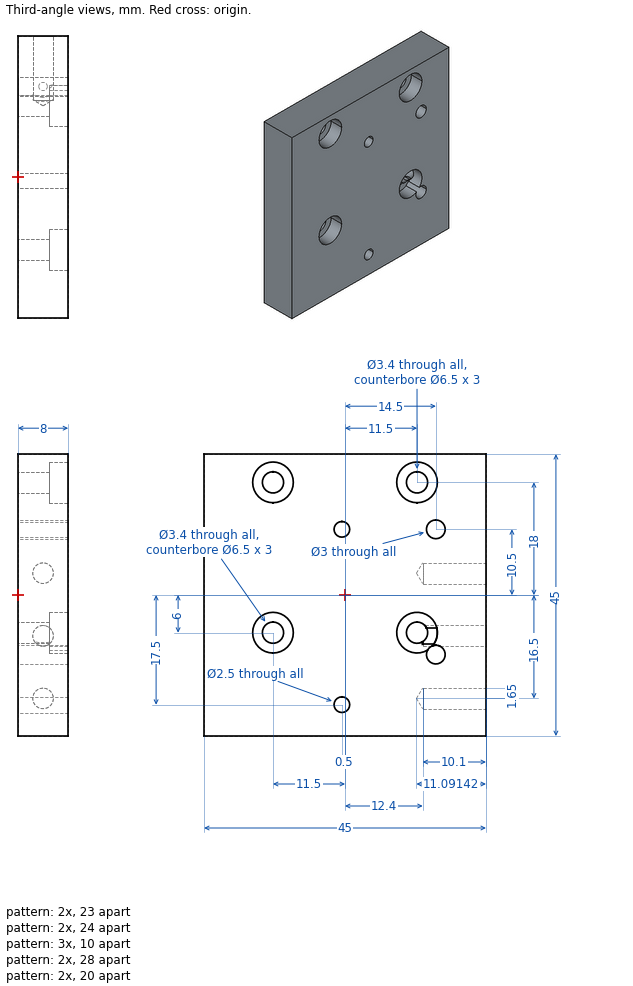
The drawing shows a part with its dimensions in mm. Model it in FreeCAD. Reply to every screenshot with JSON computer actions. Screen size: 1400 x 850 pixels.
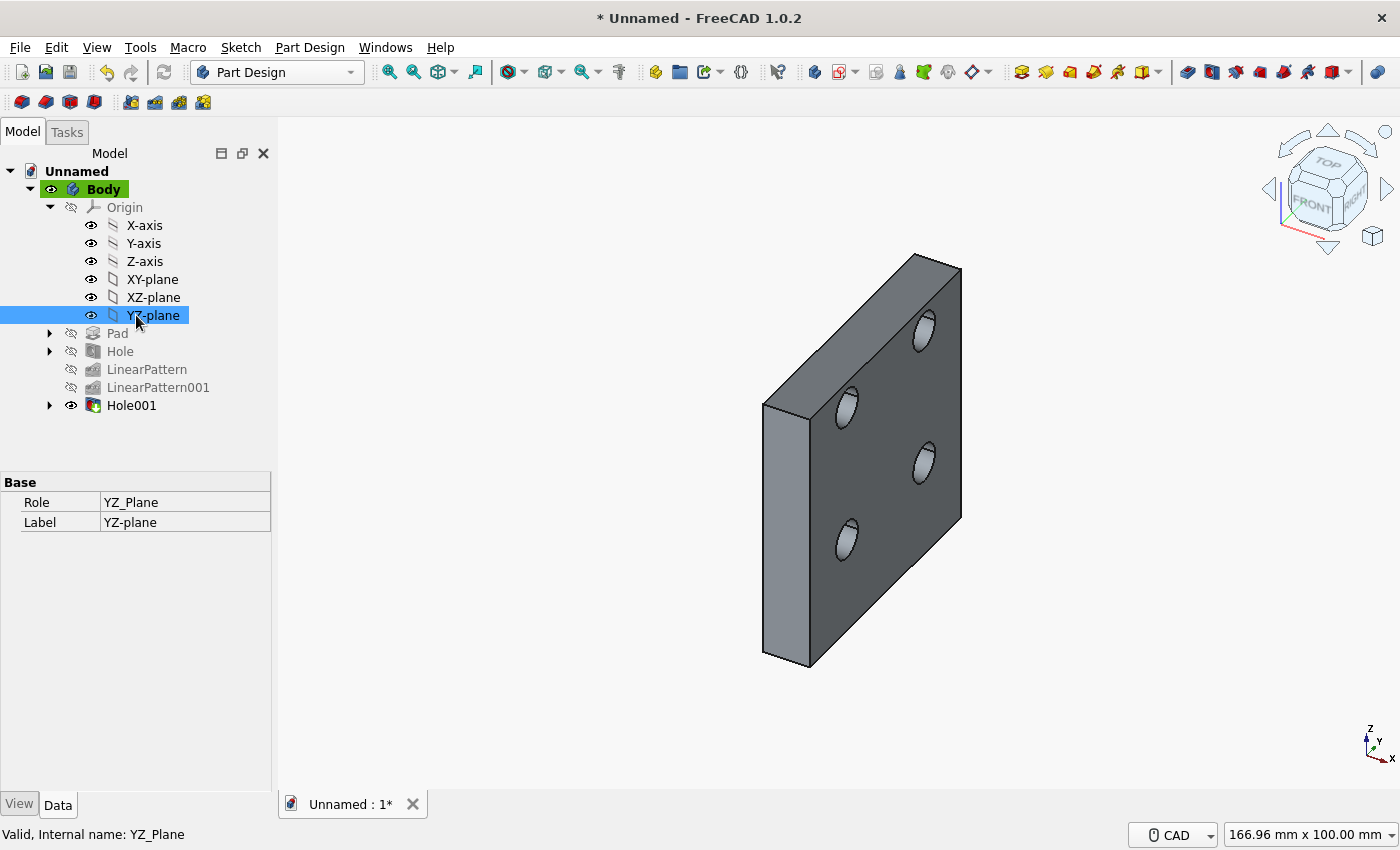
{"action": "left_click", "coordinate": [972, 72]}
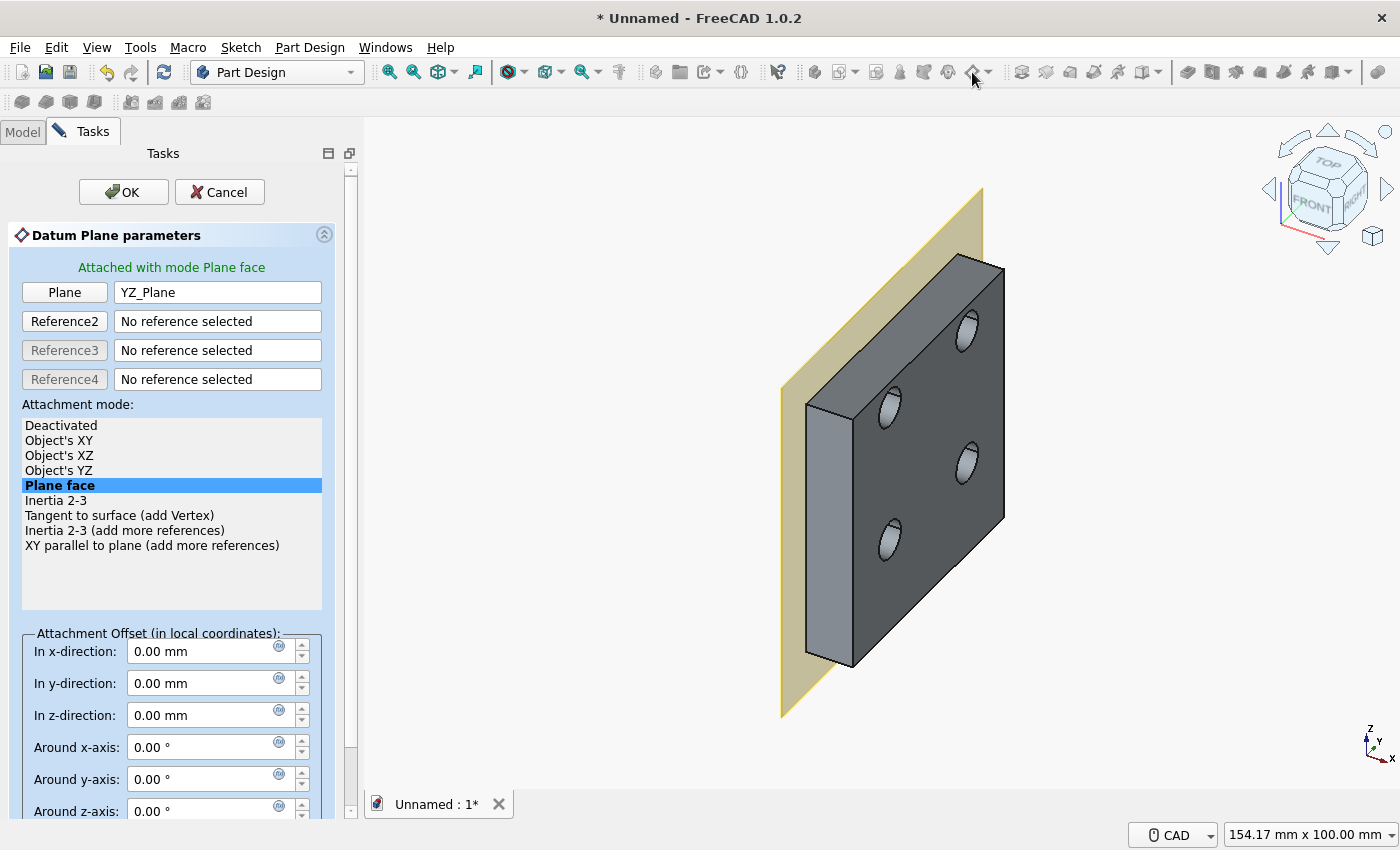
{"action": "triple_click", "coordinate": [210, 715]}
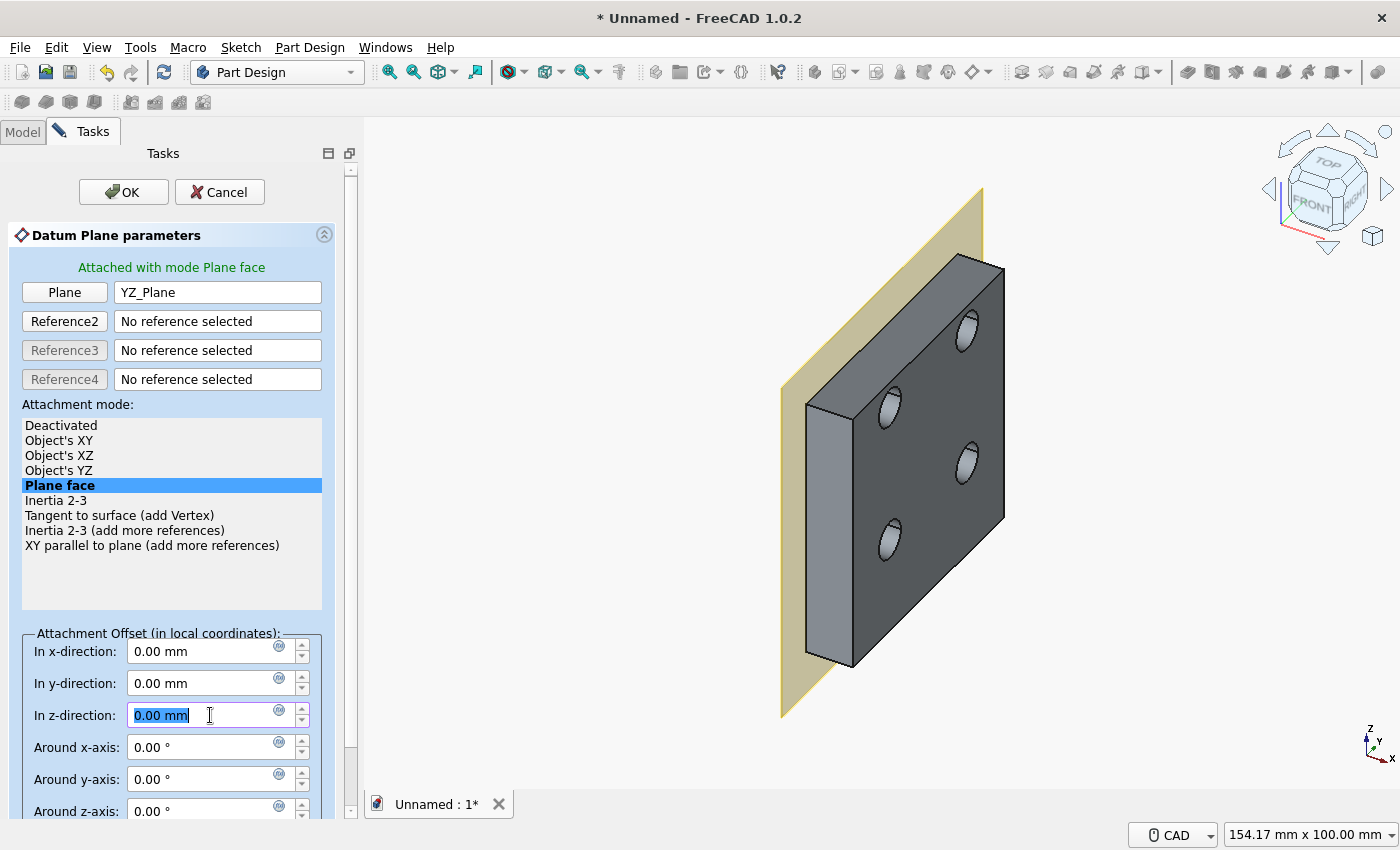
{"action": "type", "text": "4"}
{"action": "key", "text": "Tab"}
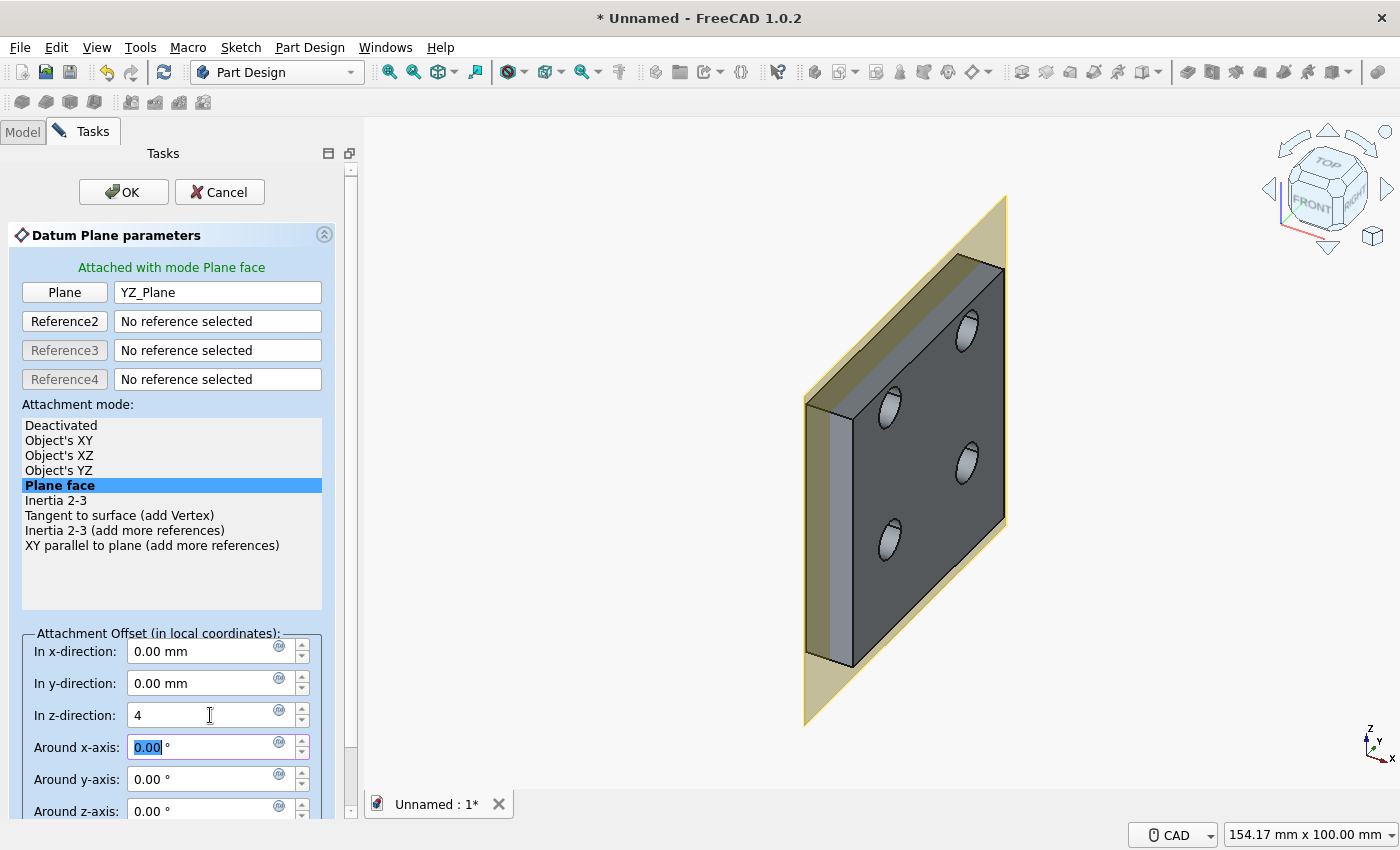
{"action": "left_click", "coordinate": [124, 192]}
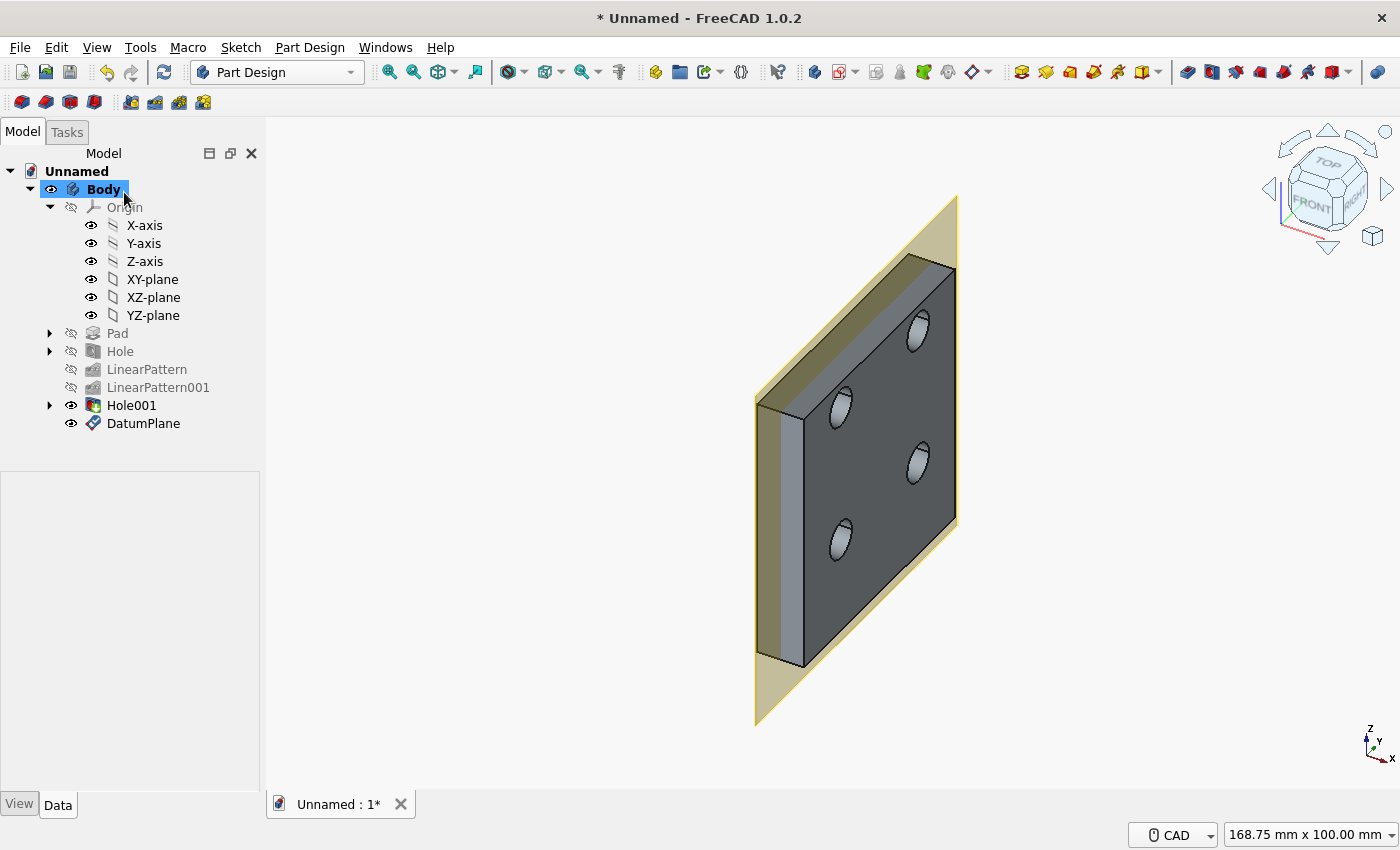
{"action": "left_click", "coordinate": [116, 423]}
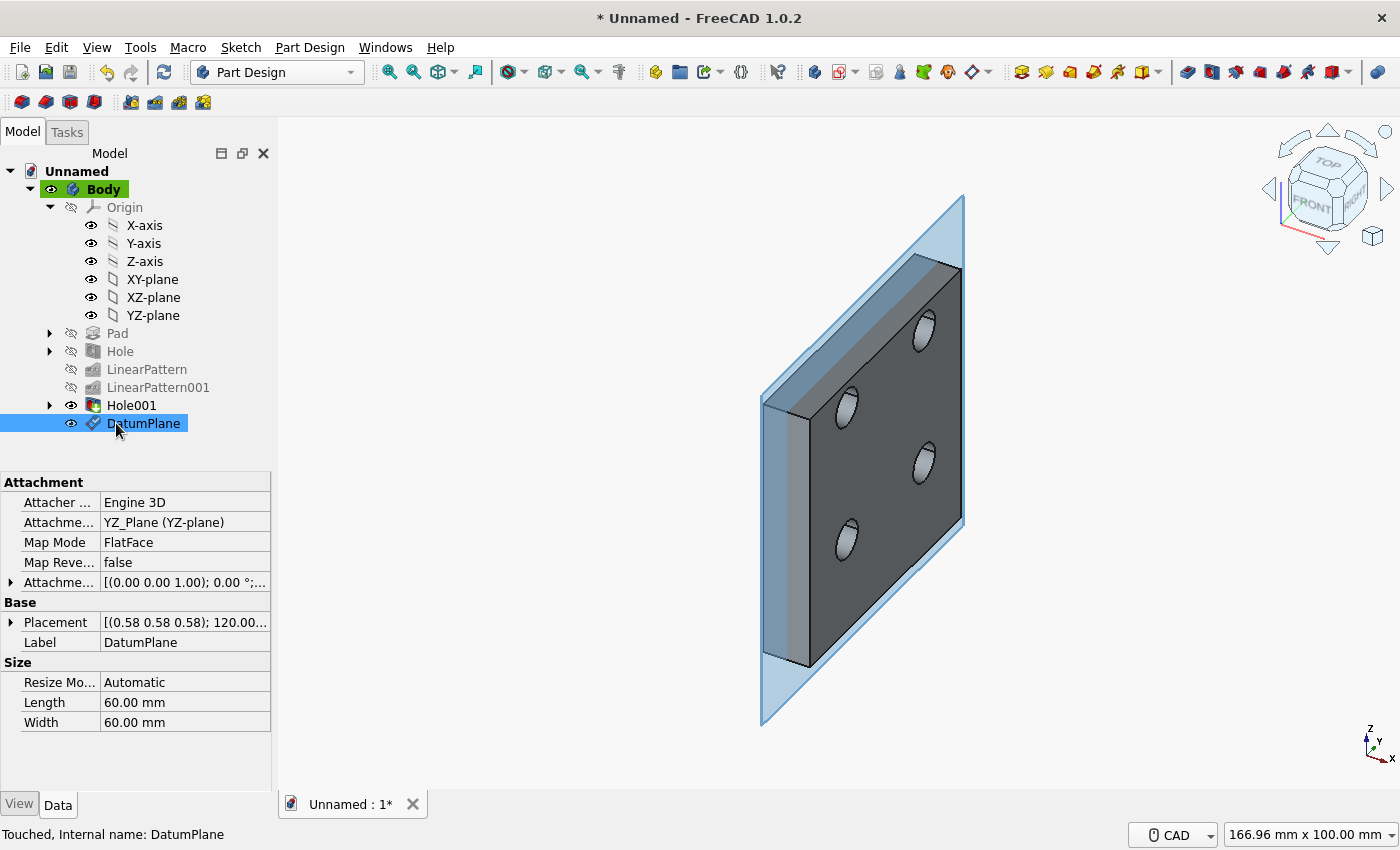
{"action": "left_click", "coordinate": [840, 72]}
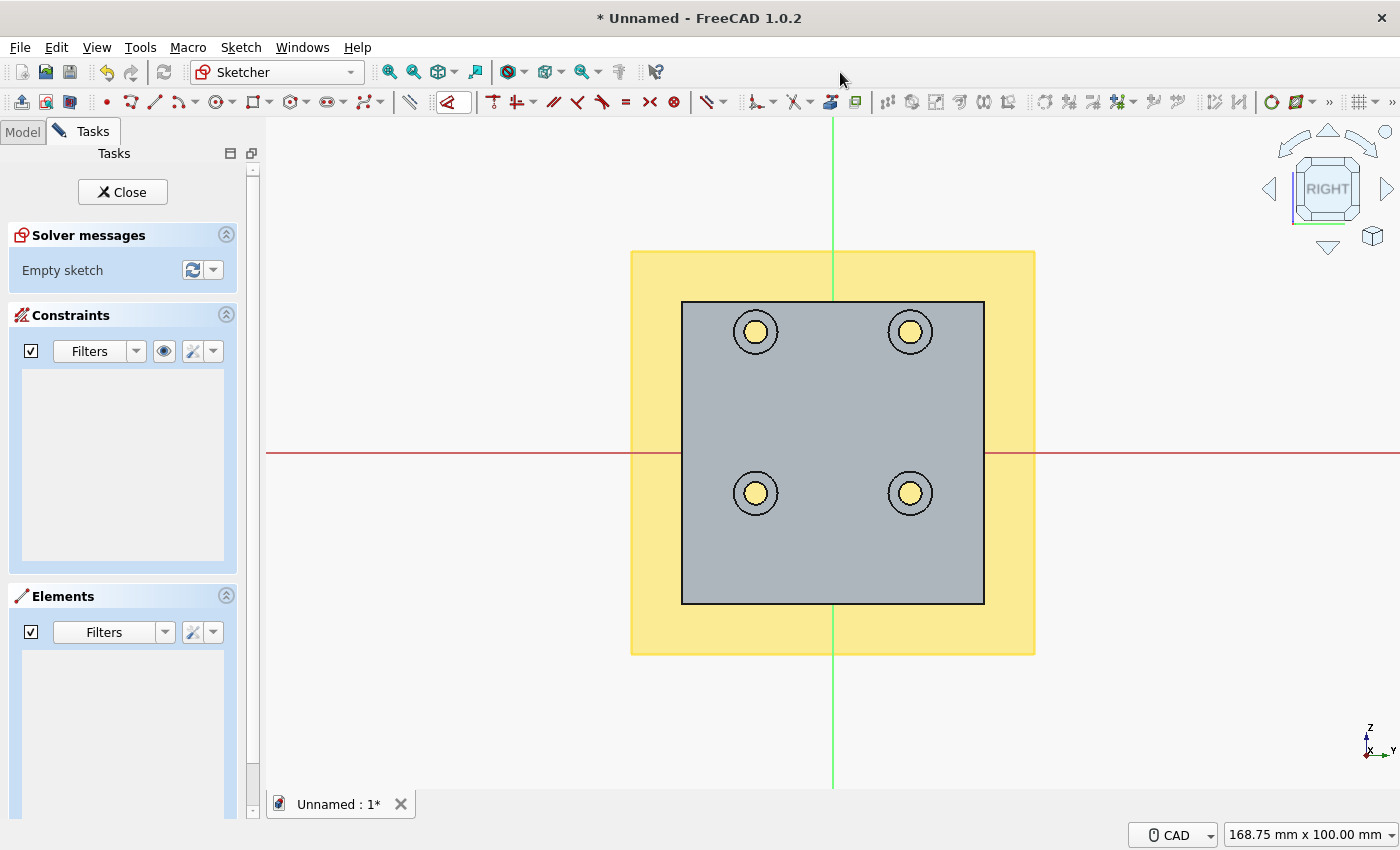
{"action": "key", "text": "q s"}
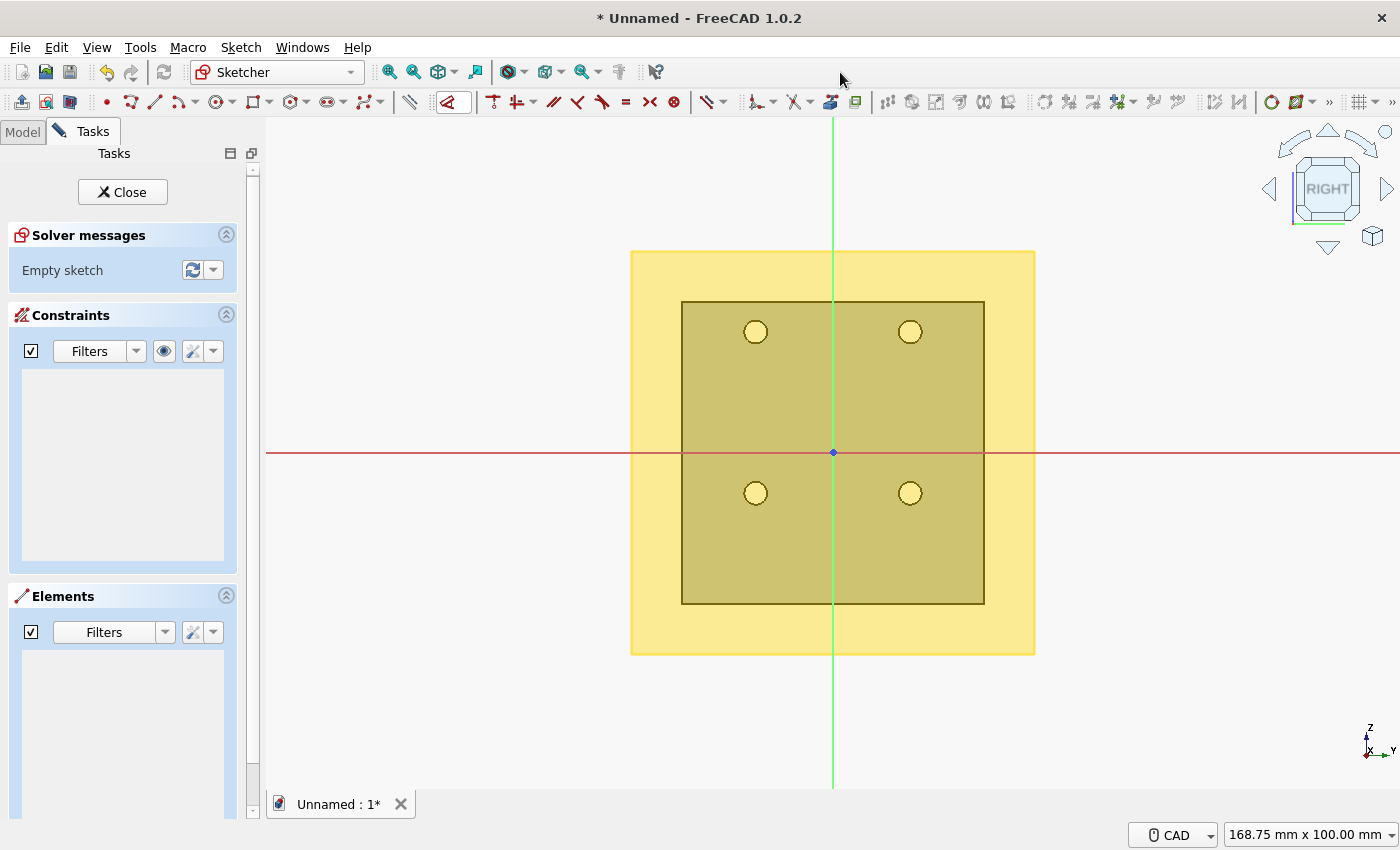
{"action": "scroll", "coordinate": [956, 527], "scroll_direction": "up", "scroll_amount": 7}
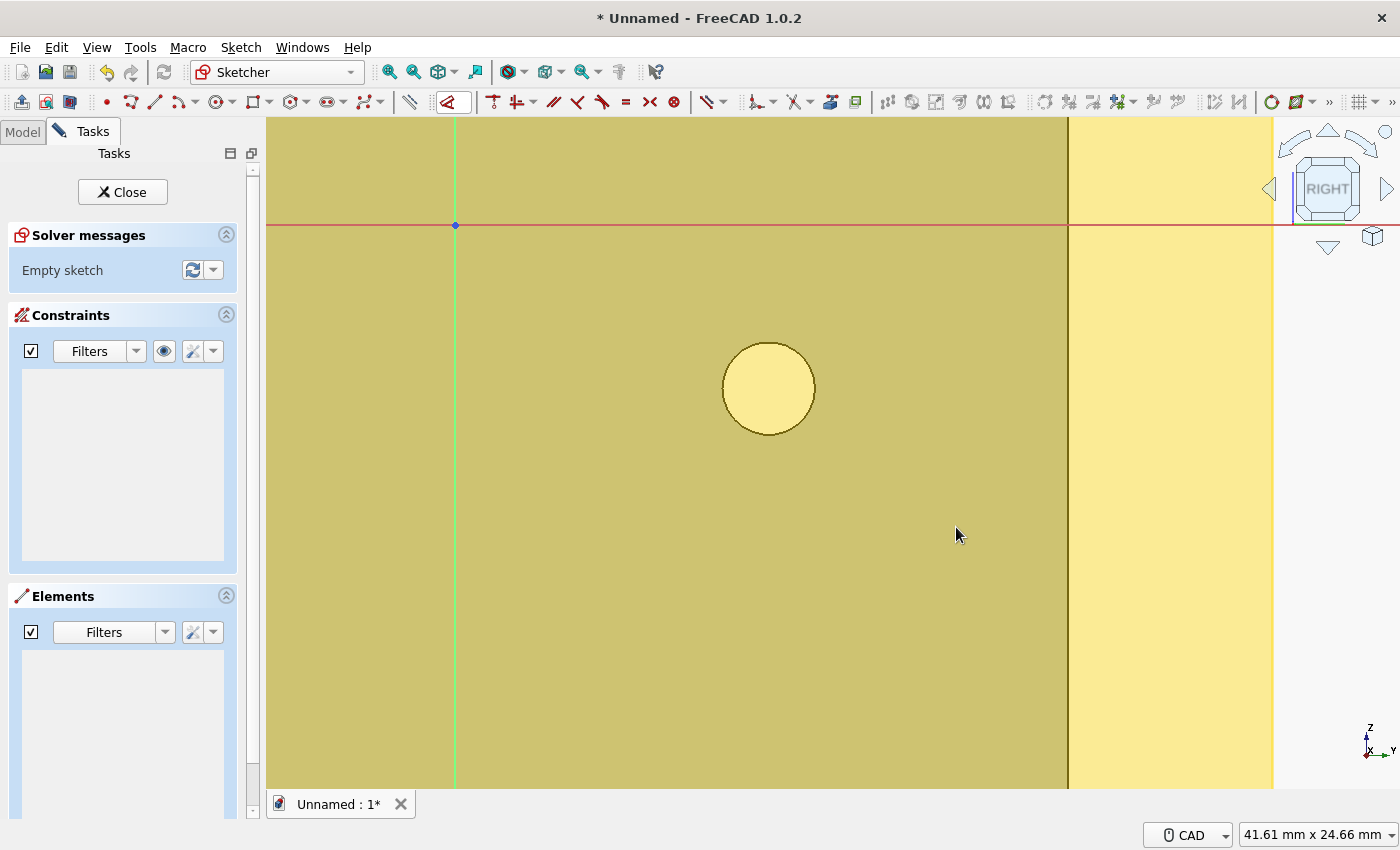
{"action": "left_click", "coordinate": [132, 102]}